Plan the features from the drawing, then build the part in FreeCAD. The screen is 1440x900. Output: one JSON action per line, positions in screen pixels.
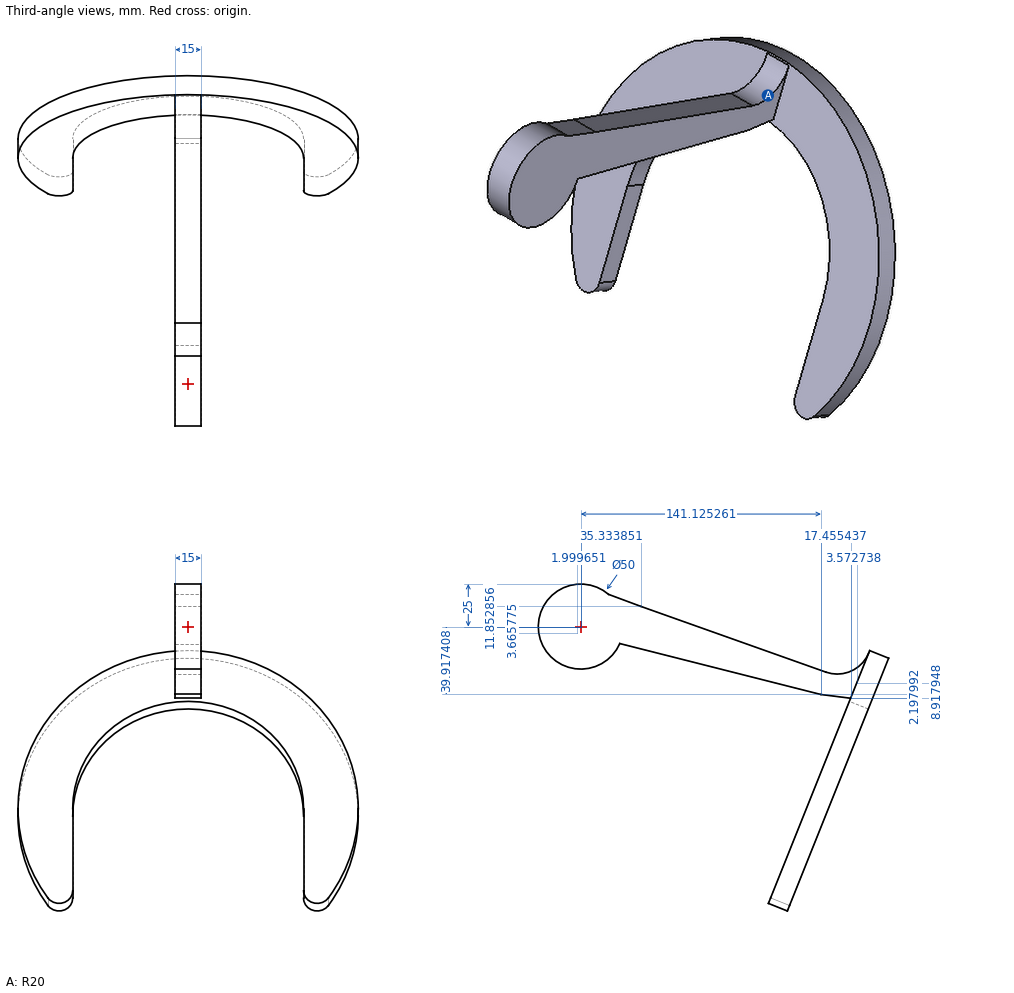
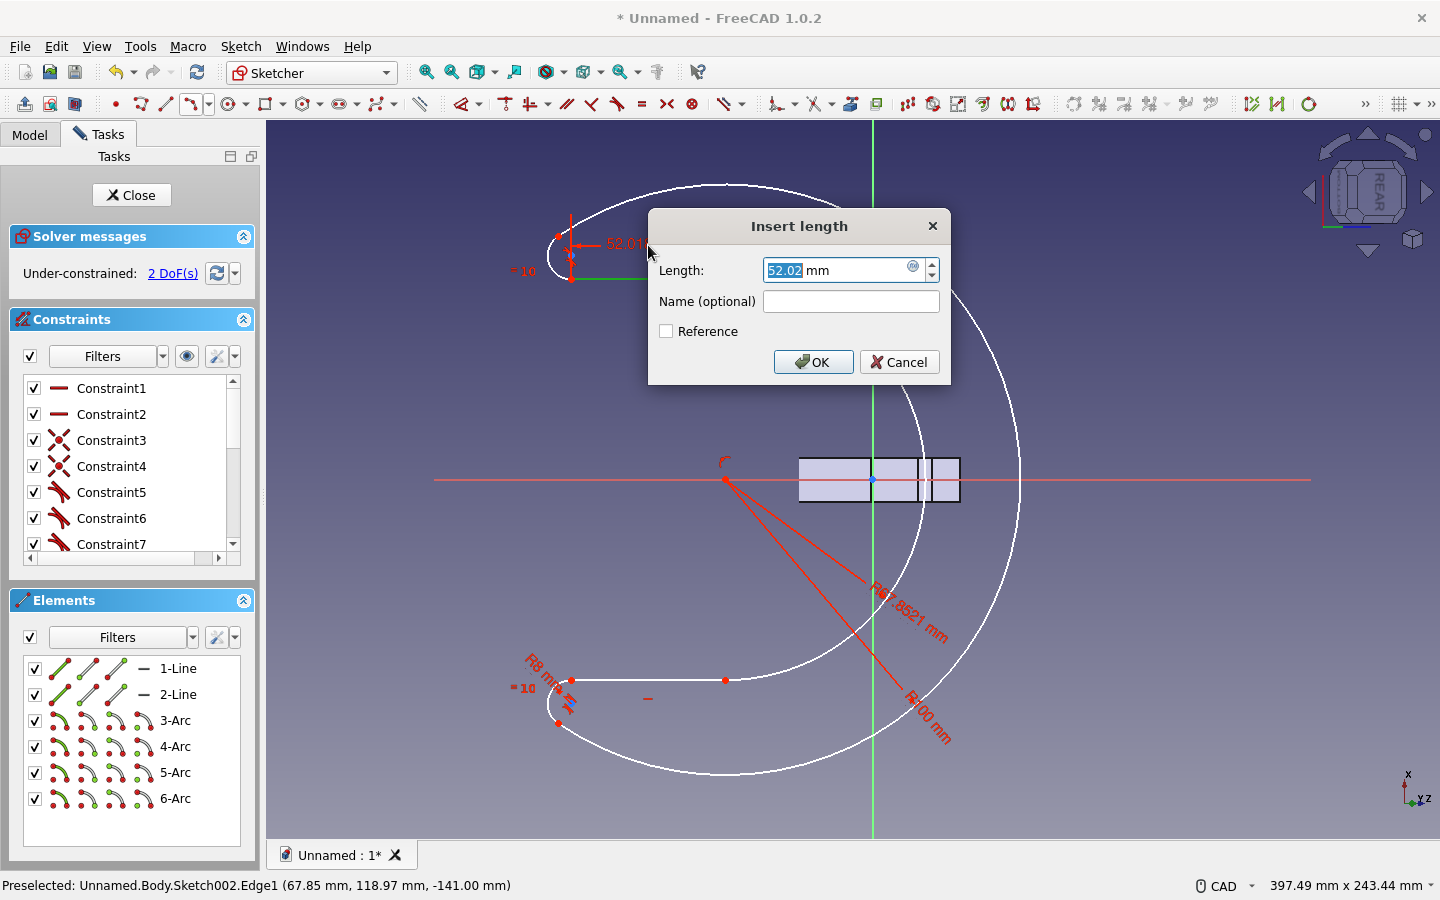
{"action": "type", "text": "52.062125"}
{"action": "key", "text": "Return"}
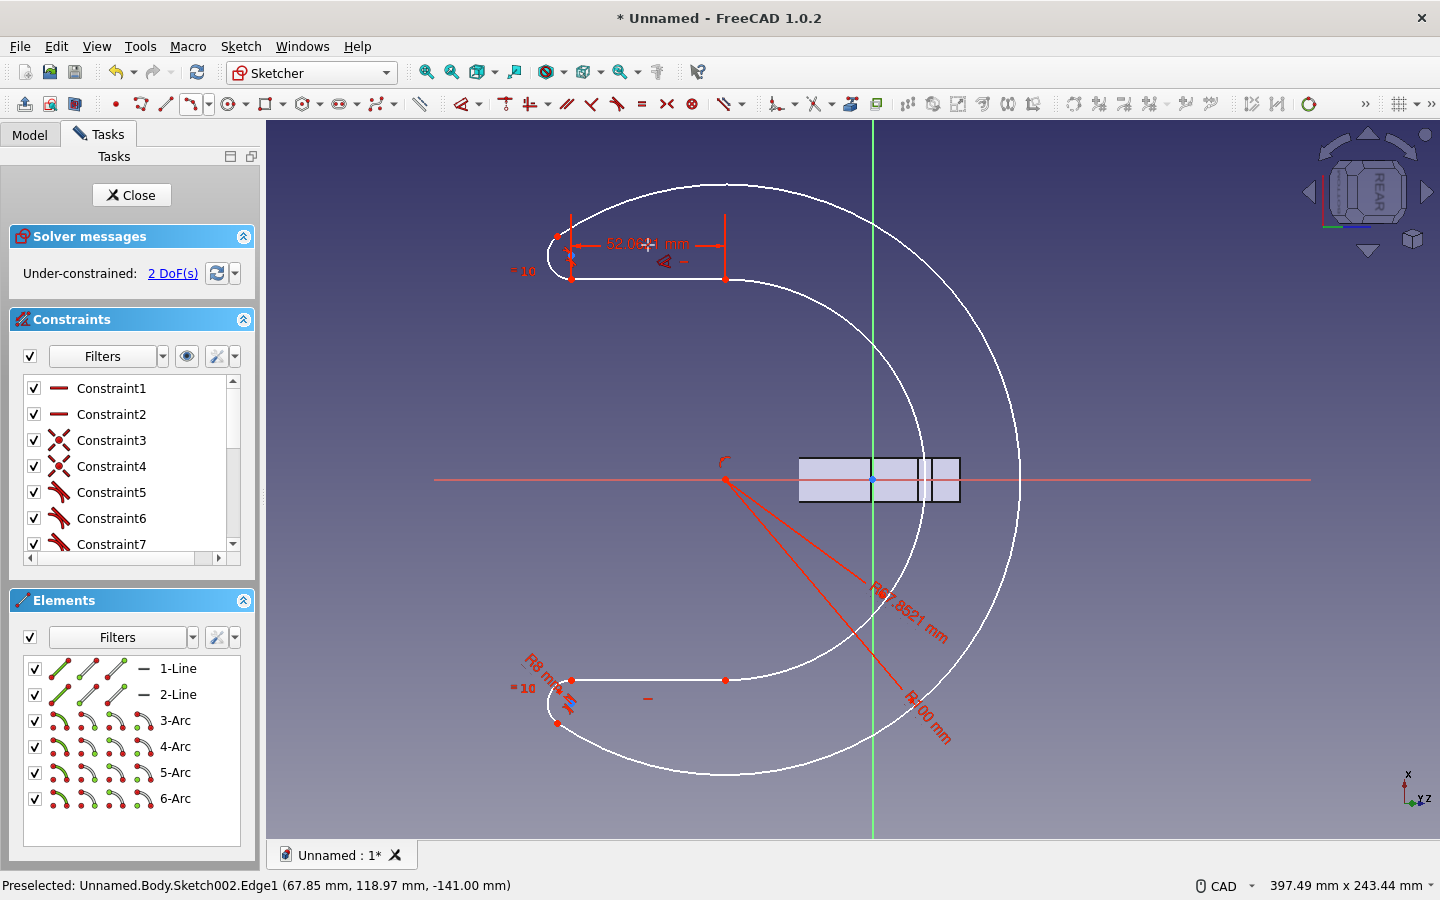
{"action": "left_click", "coordinate": [679, 680]}
{"action": "left_click", "coordinate": [648, 714]}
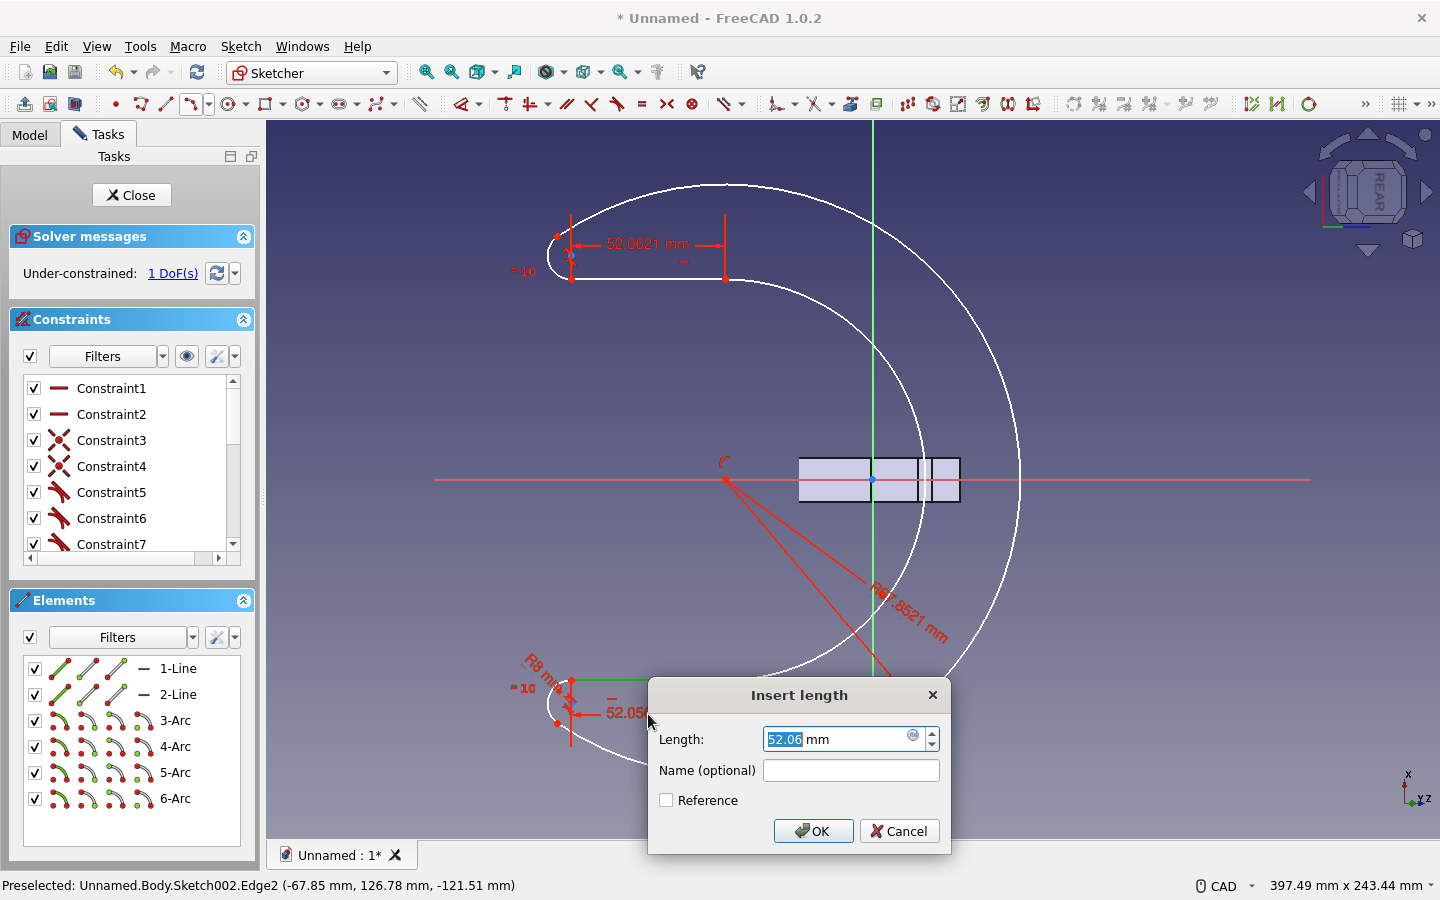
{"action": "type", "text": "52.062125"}
{"action": "key", "text": "Return"}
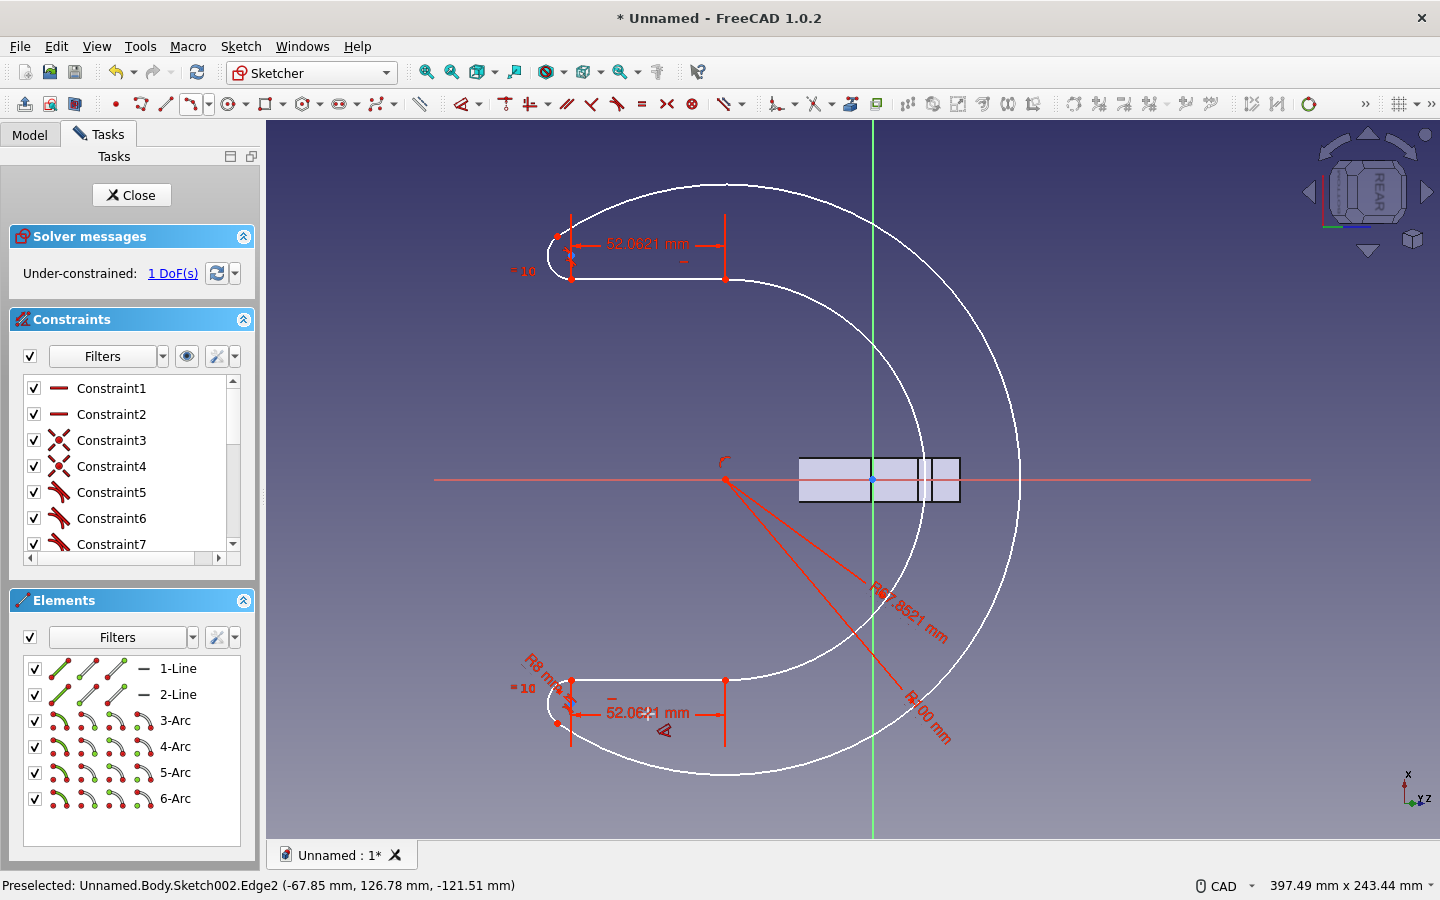
{"action": "left_click", "coordinate": [725, 279]}
{"action": "left_click", "coordinate": [799, 245]}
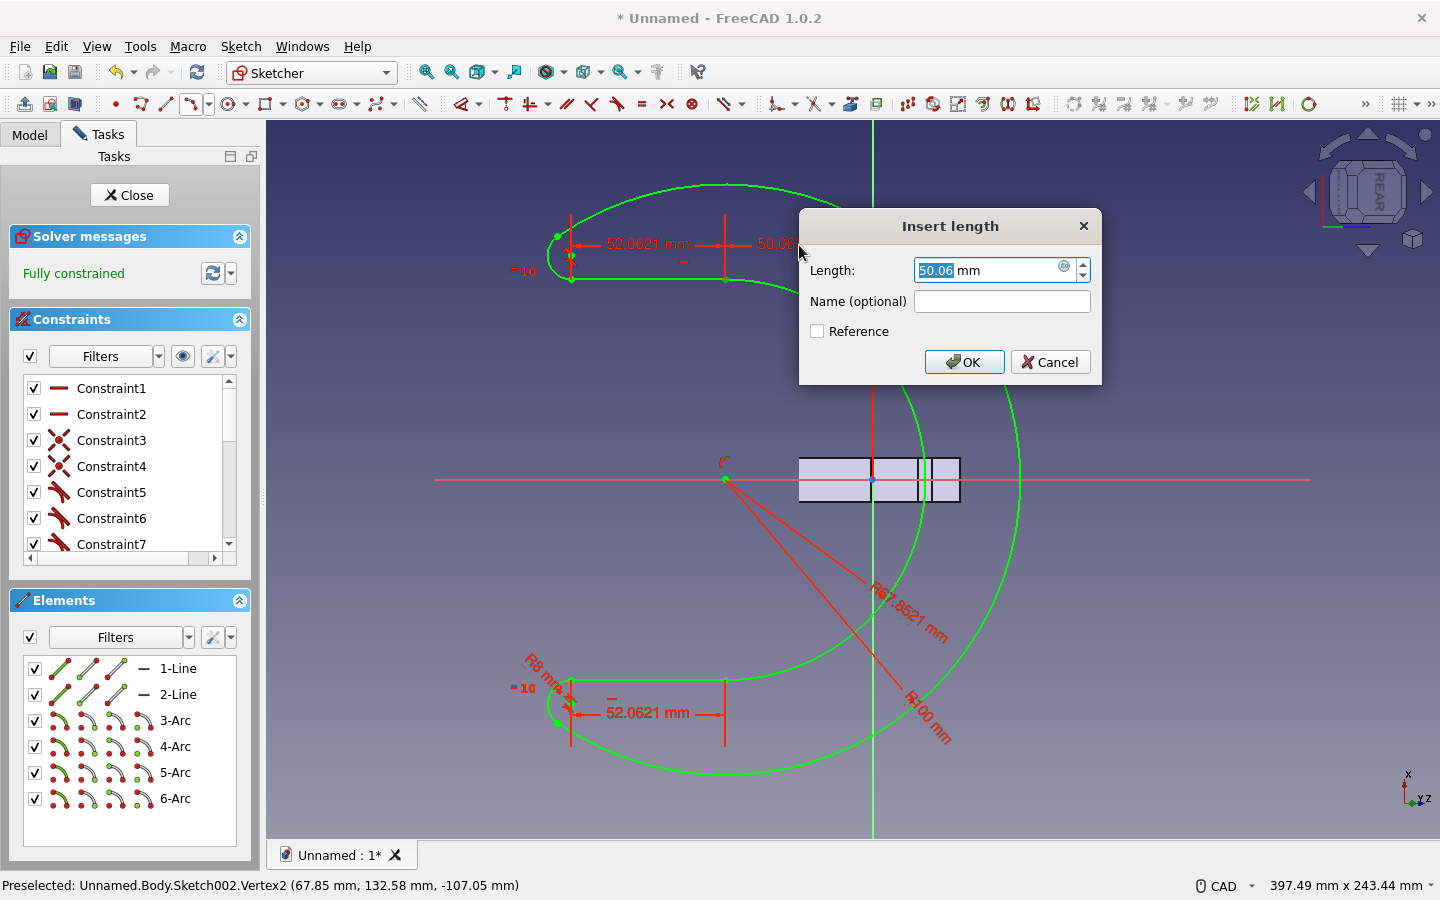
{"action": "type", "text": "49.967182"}
{"action": "key", "text": "Return"}
{"action": "key", "text": "Escape"}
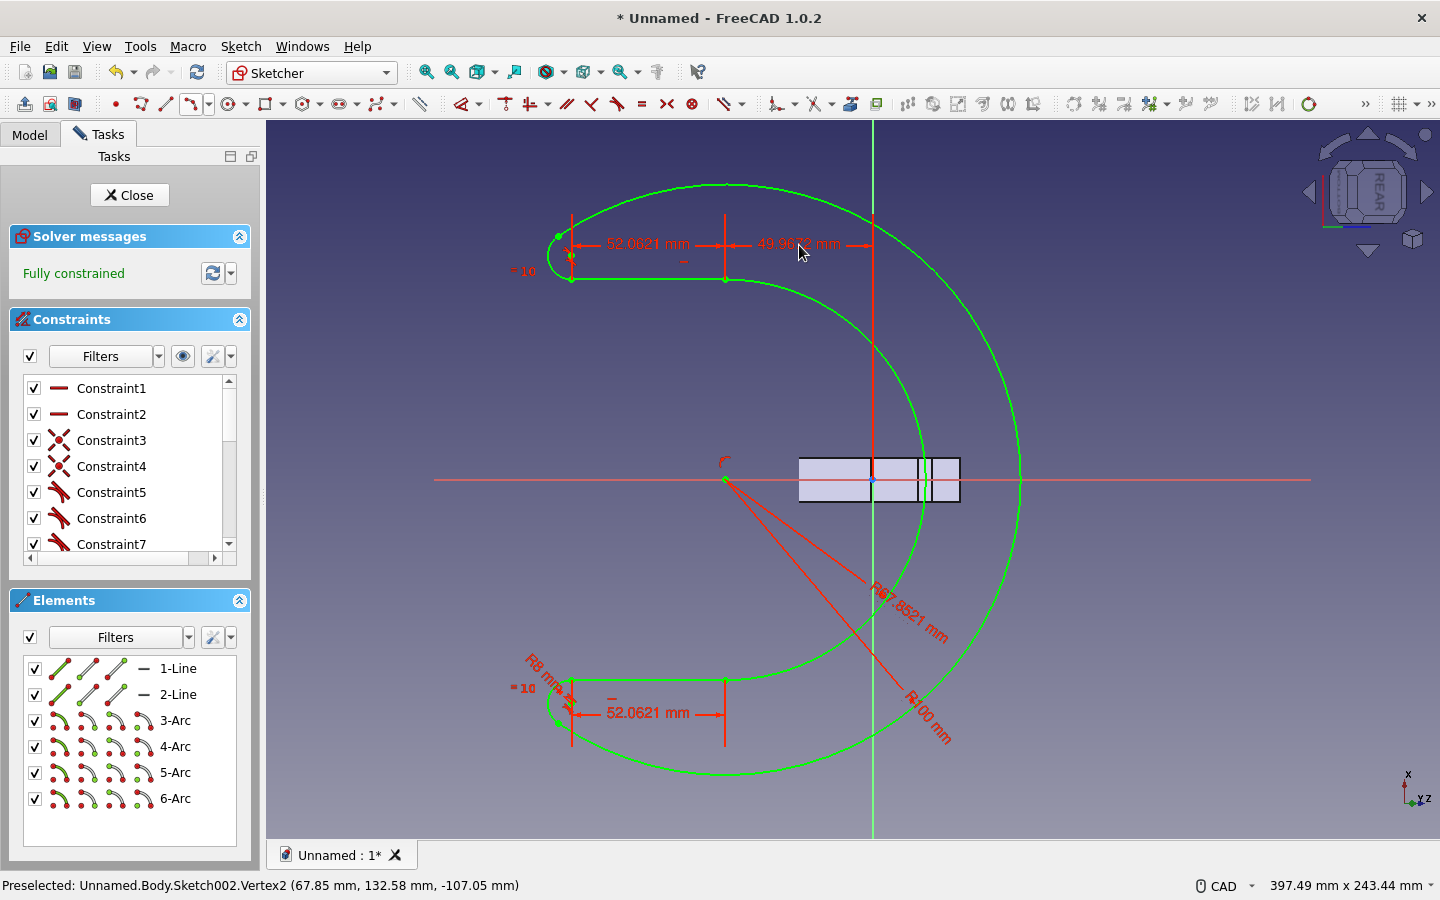
{"action": "left_click", "coordinate": [130, 195]}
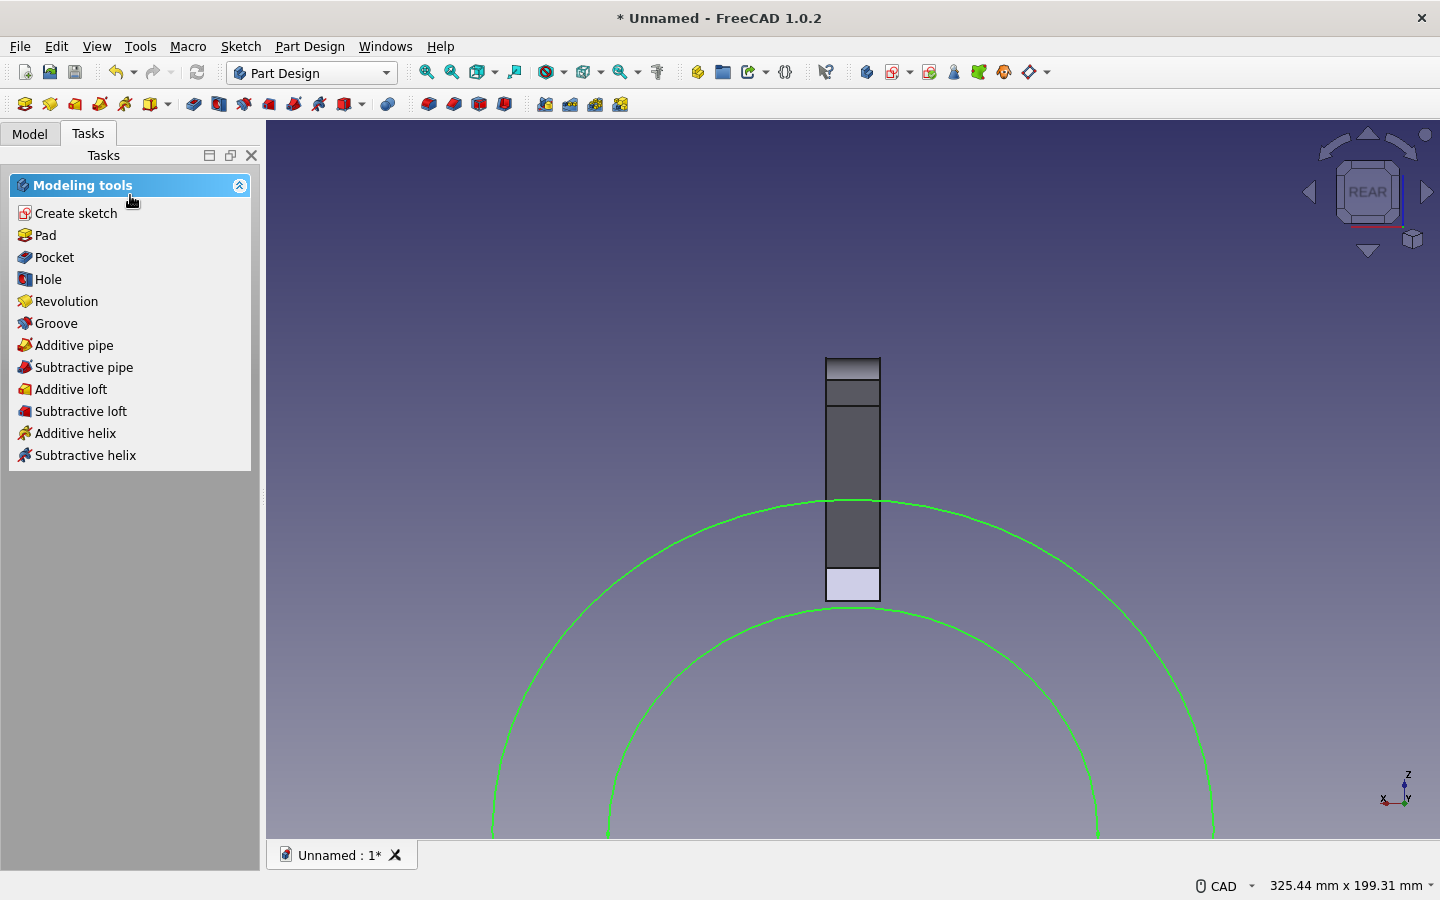
{"action": "left_click", "coordinate": [25, 104]}